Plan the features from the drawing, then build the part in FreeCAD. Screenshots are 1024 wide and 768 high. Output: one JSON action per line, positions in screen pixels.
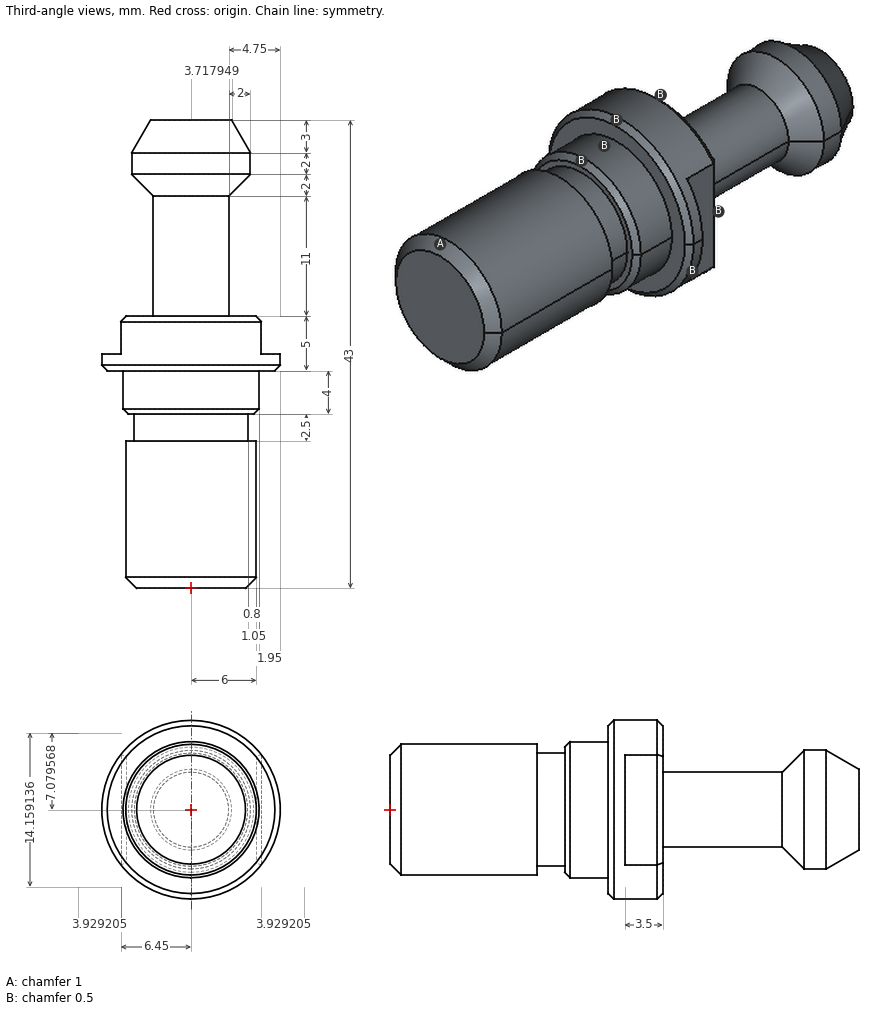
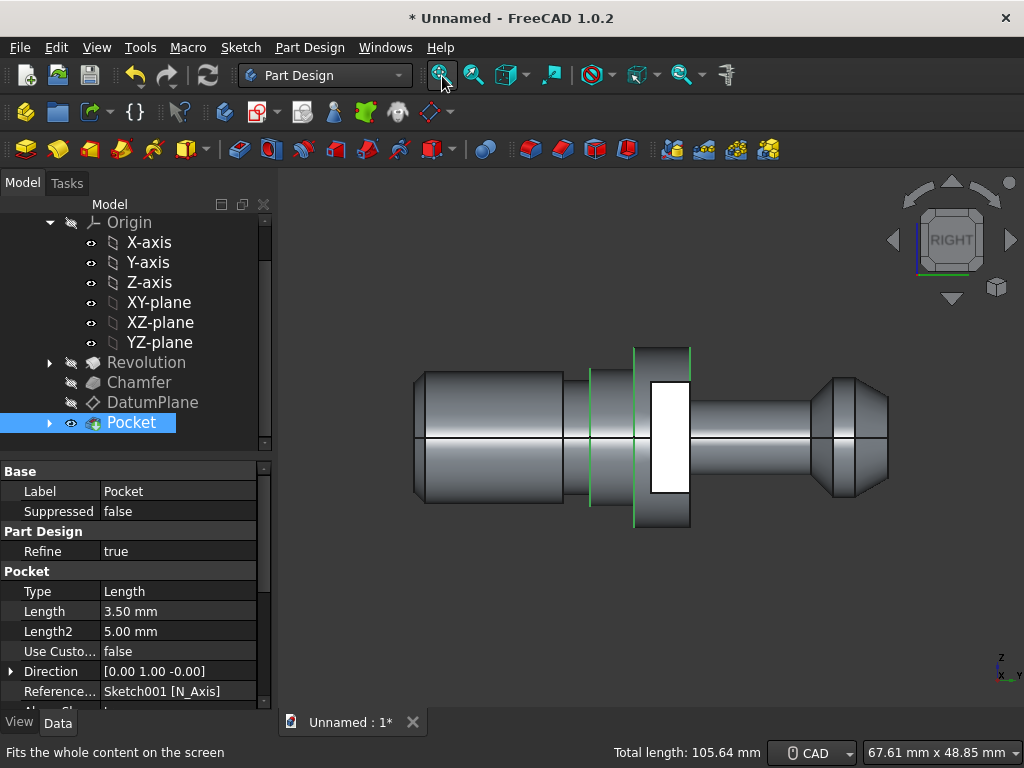
{"action": "left_click", "coordinate": [690, 436], "text": "ctrl"}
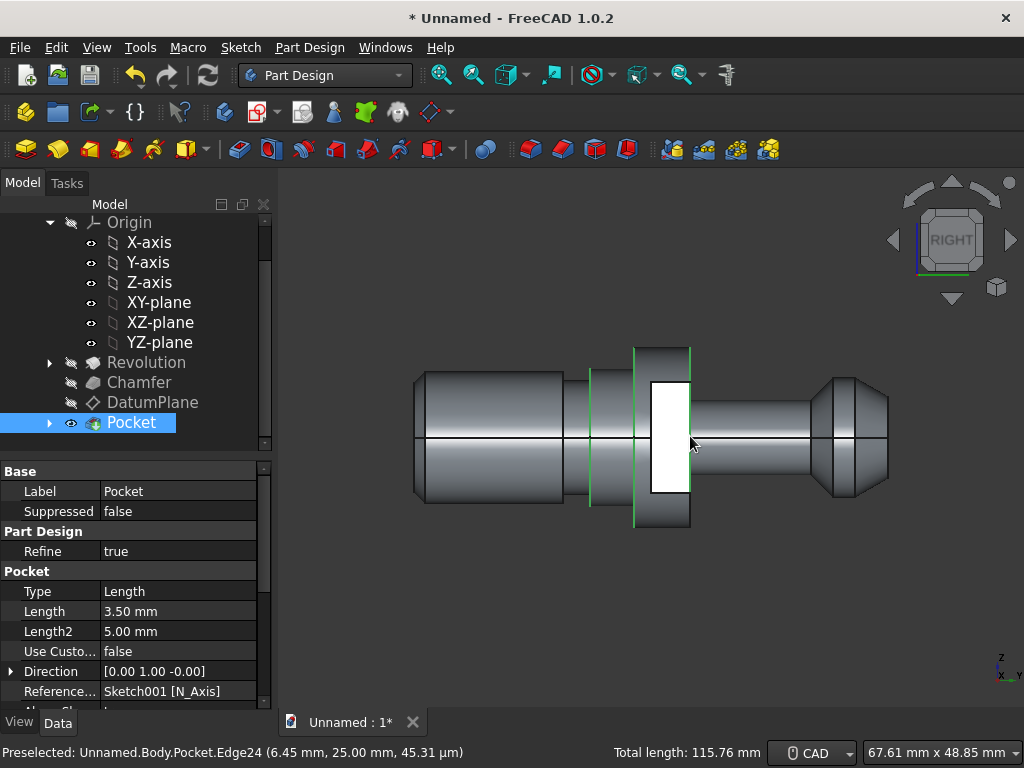
{"action": "key", "text": "5"}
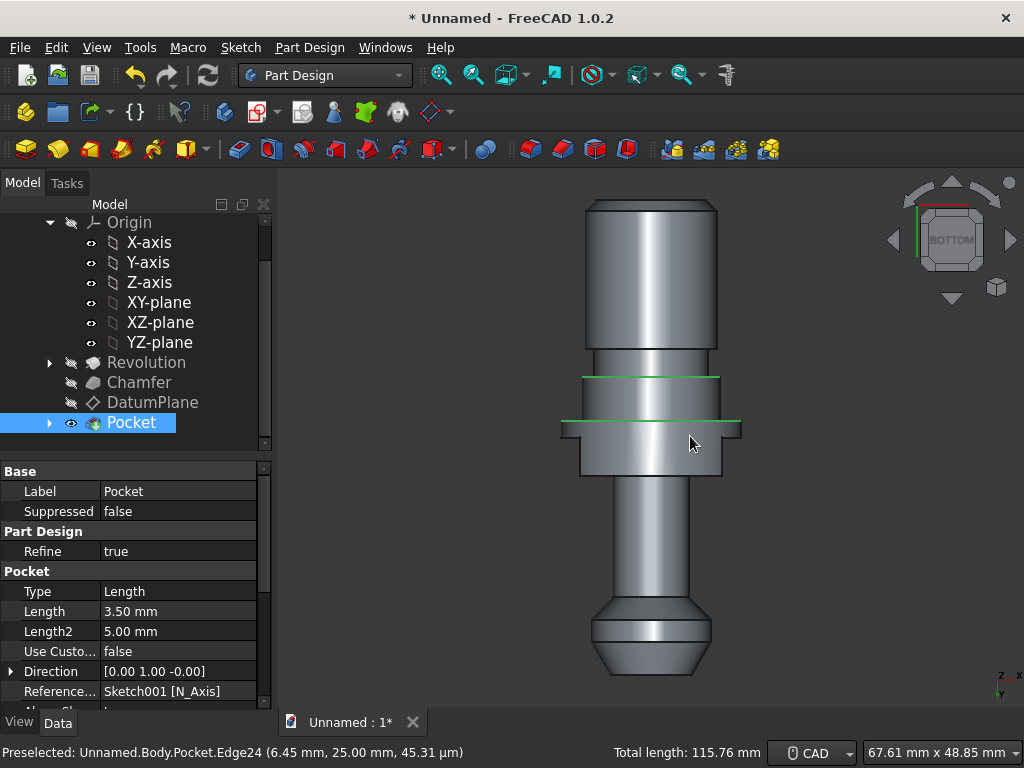
{"action": "left_click", "coordinate": [651, 475], "text": "ctrl"}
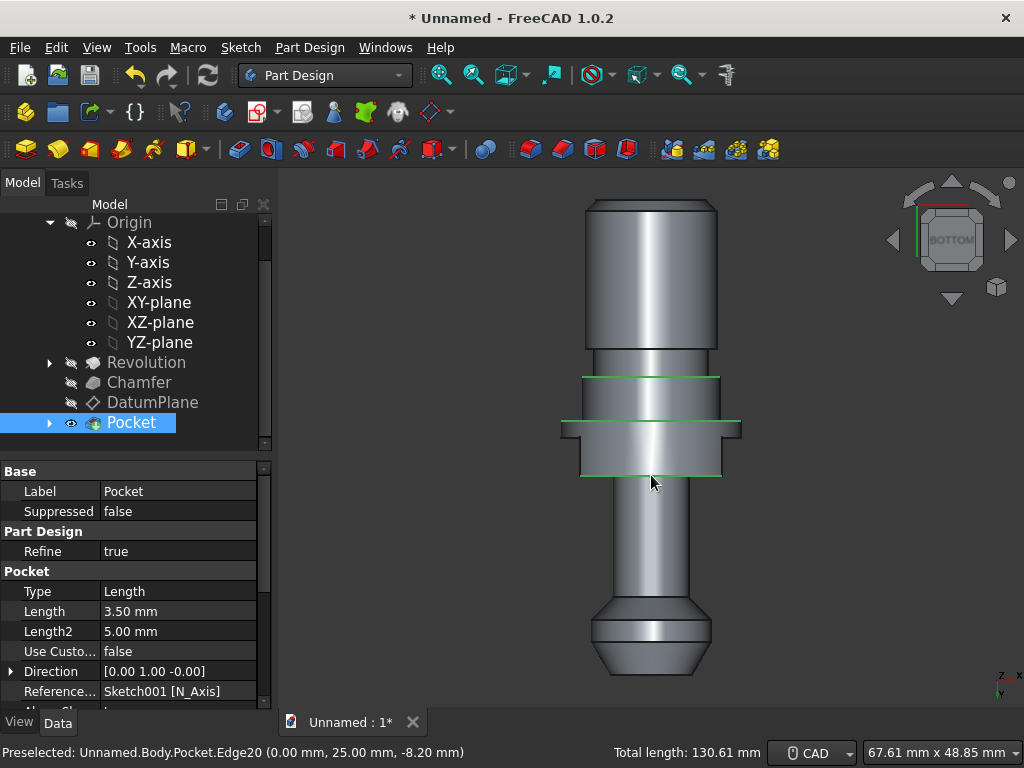
{"action": "key", "text": "4"}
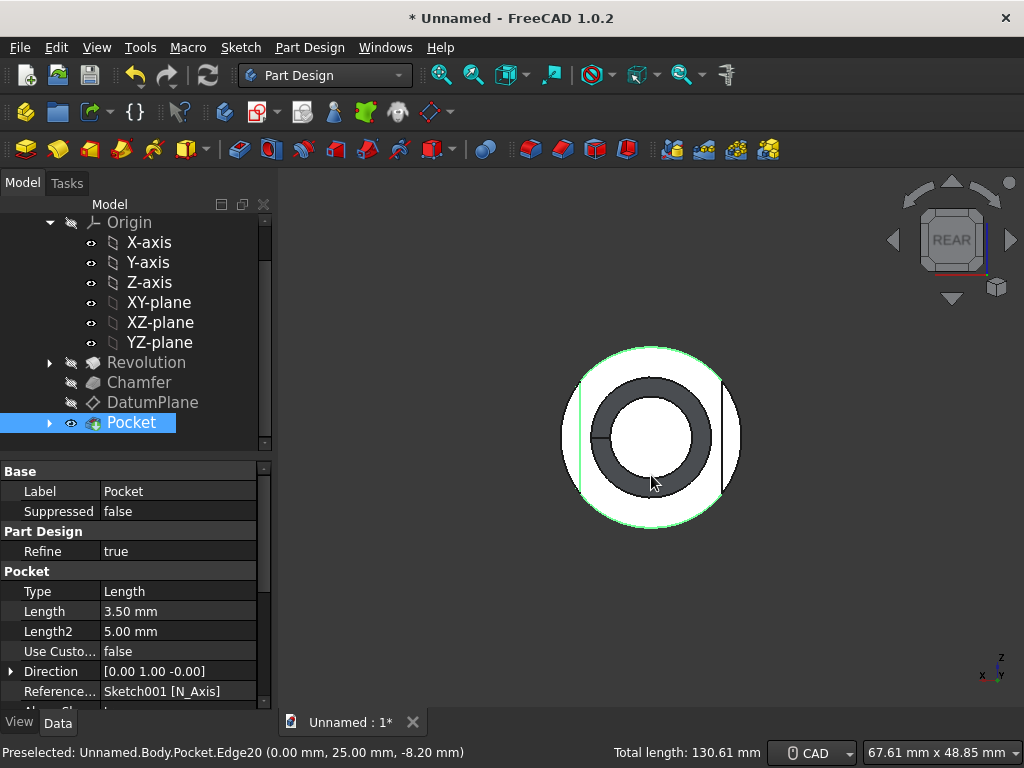
{"action": "left_click", "coordinate": [442, 76]}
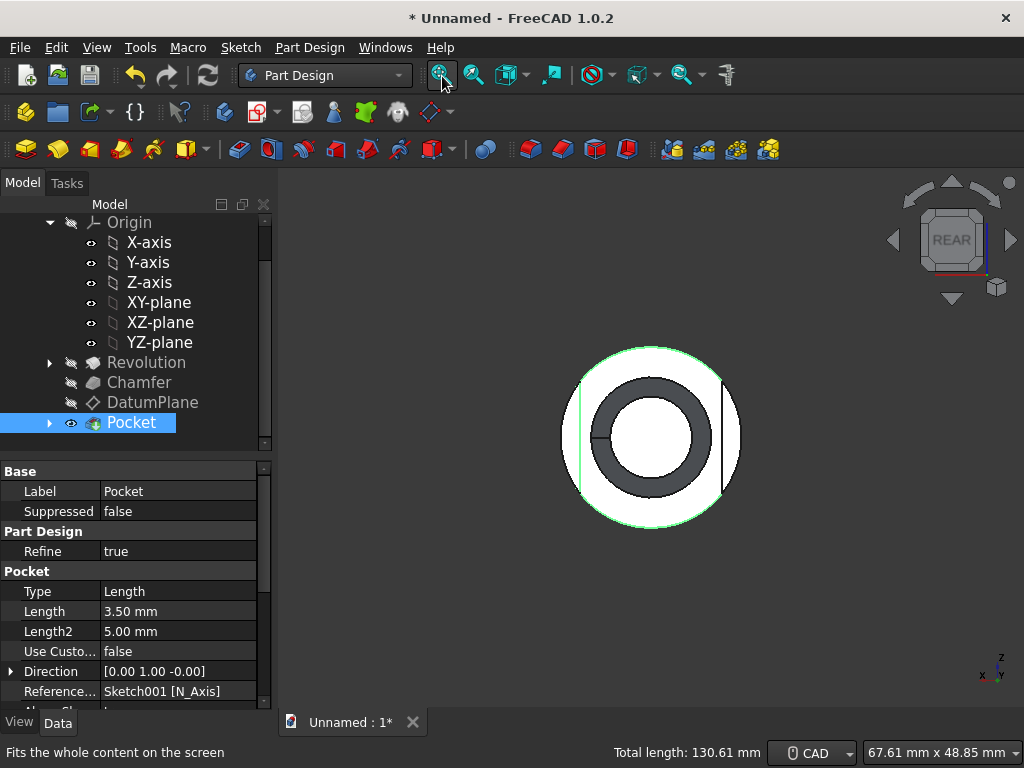
{"action": "left_click", "coordinate": [722, 437], "text": "ctrl"}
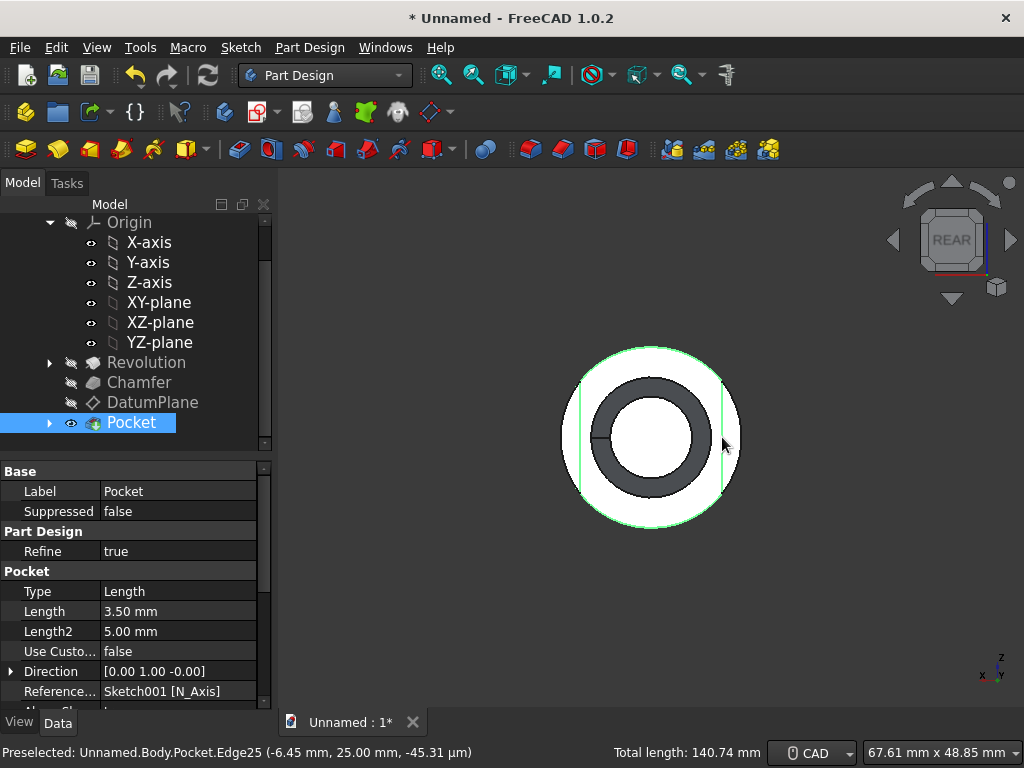
{"action": "left_click", "coordinate": [564, 150]}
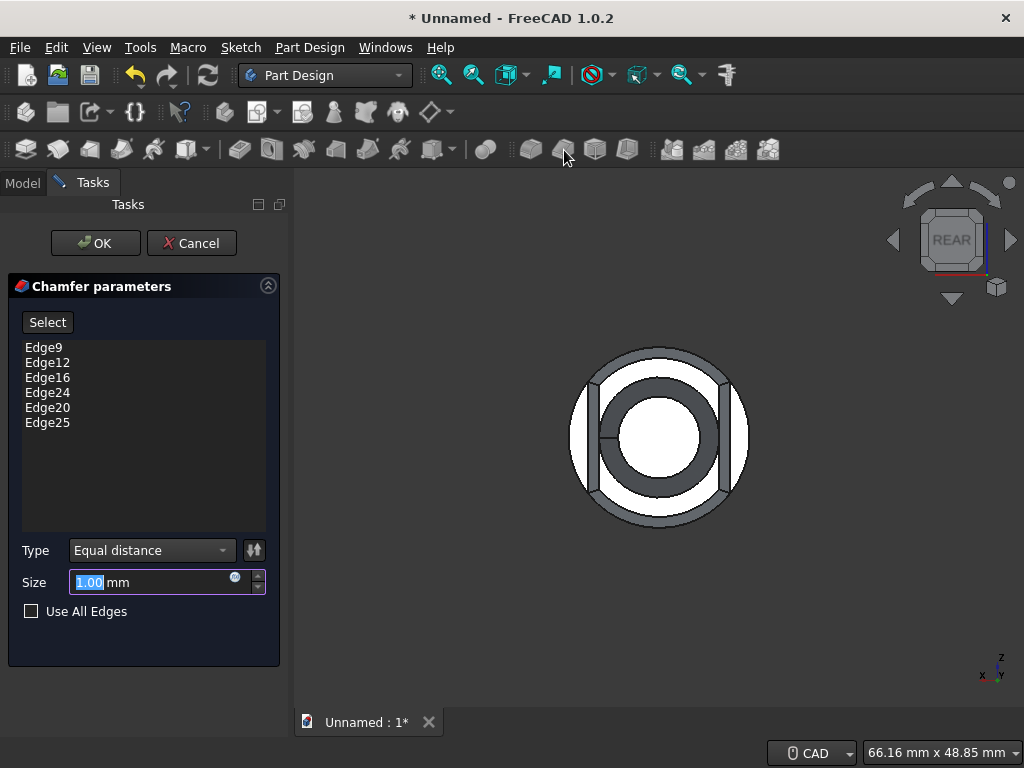
{"action": "type", "text": "0.5"}
{"action": "key", "text": "Tab"}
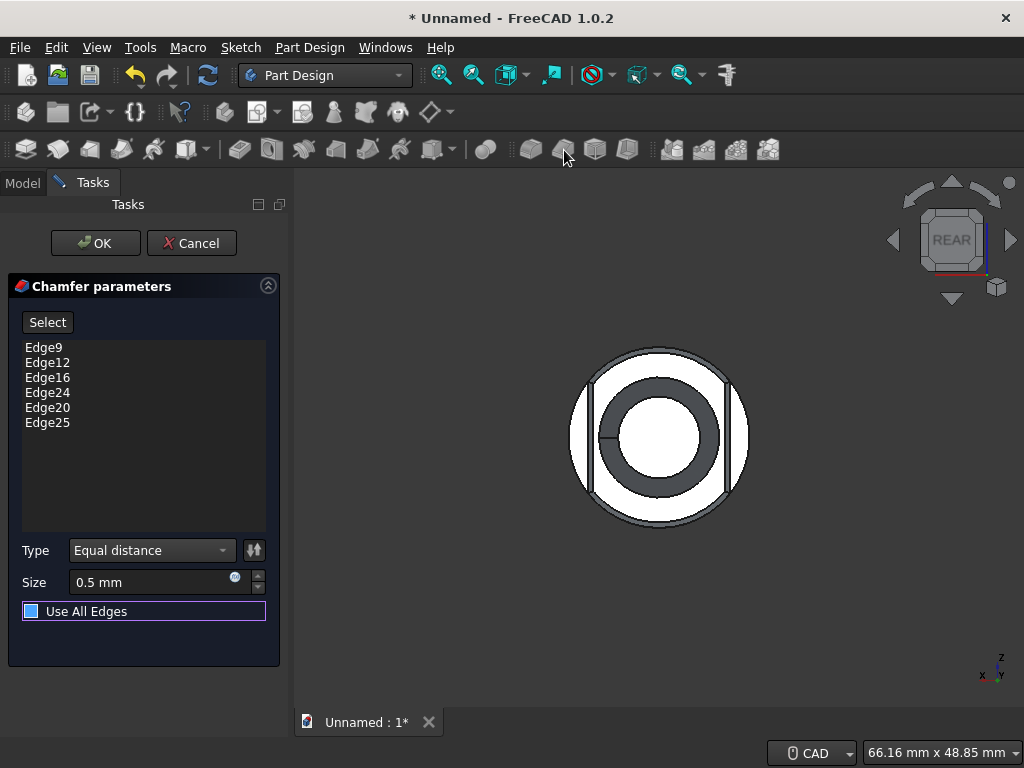
{"action": "left_click", "coordinate": [96, 243]}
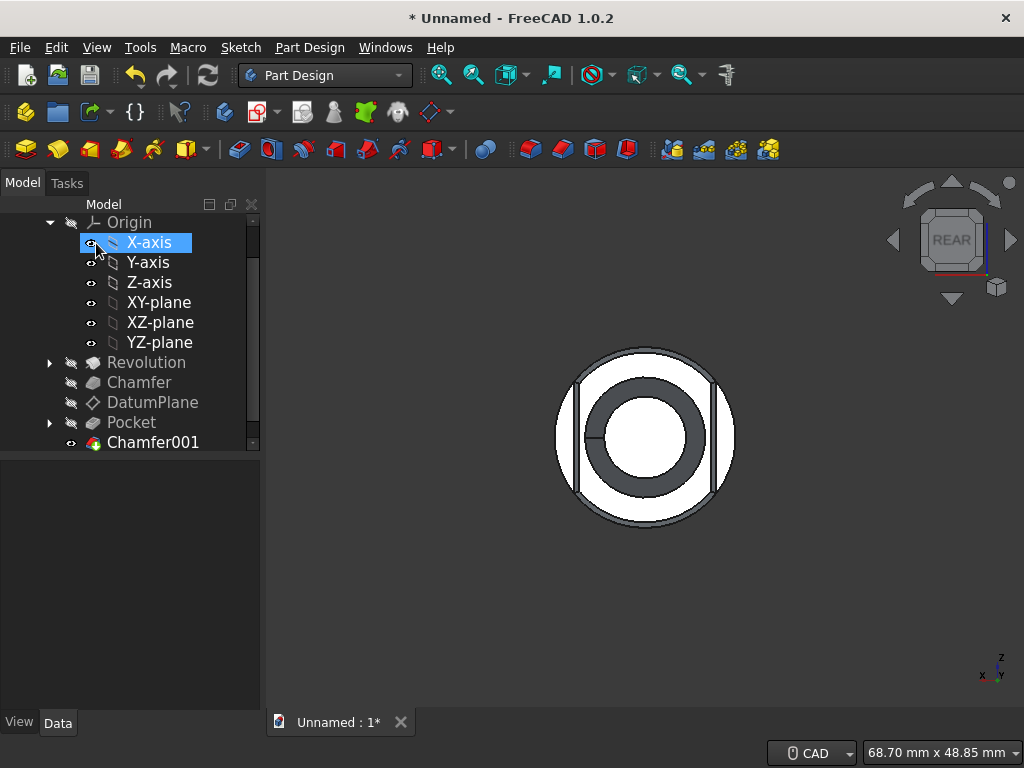
{"action": "key", "text": "0"}